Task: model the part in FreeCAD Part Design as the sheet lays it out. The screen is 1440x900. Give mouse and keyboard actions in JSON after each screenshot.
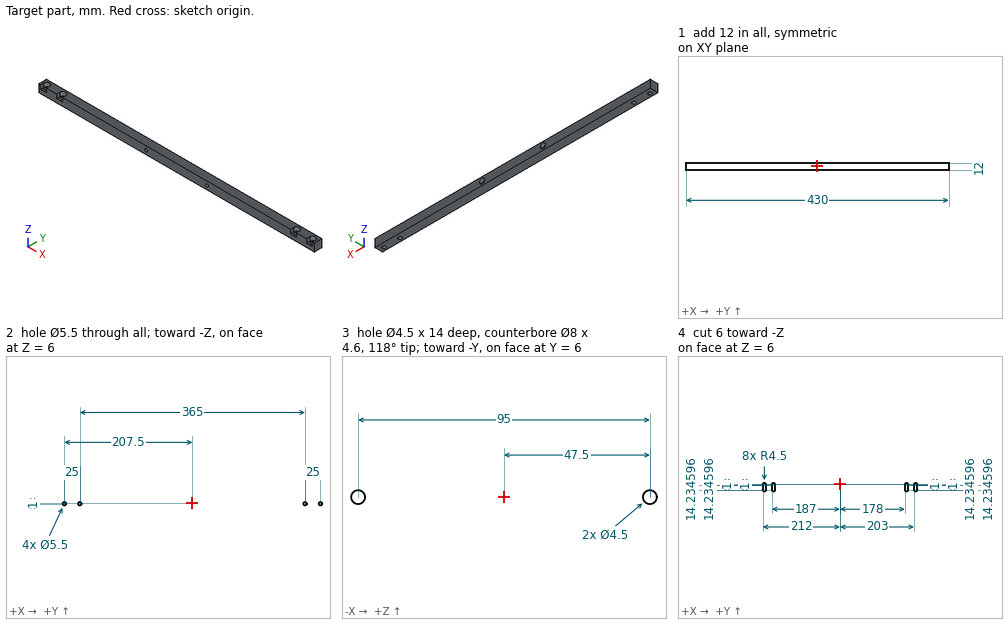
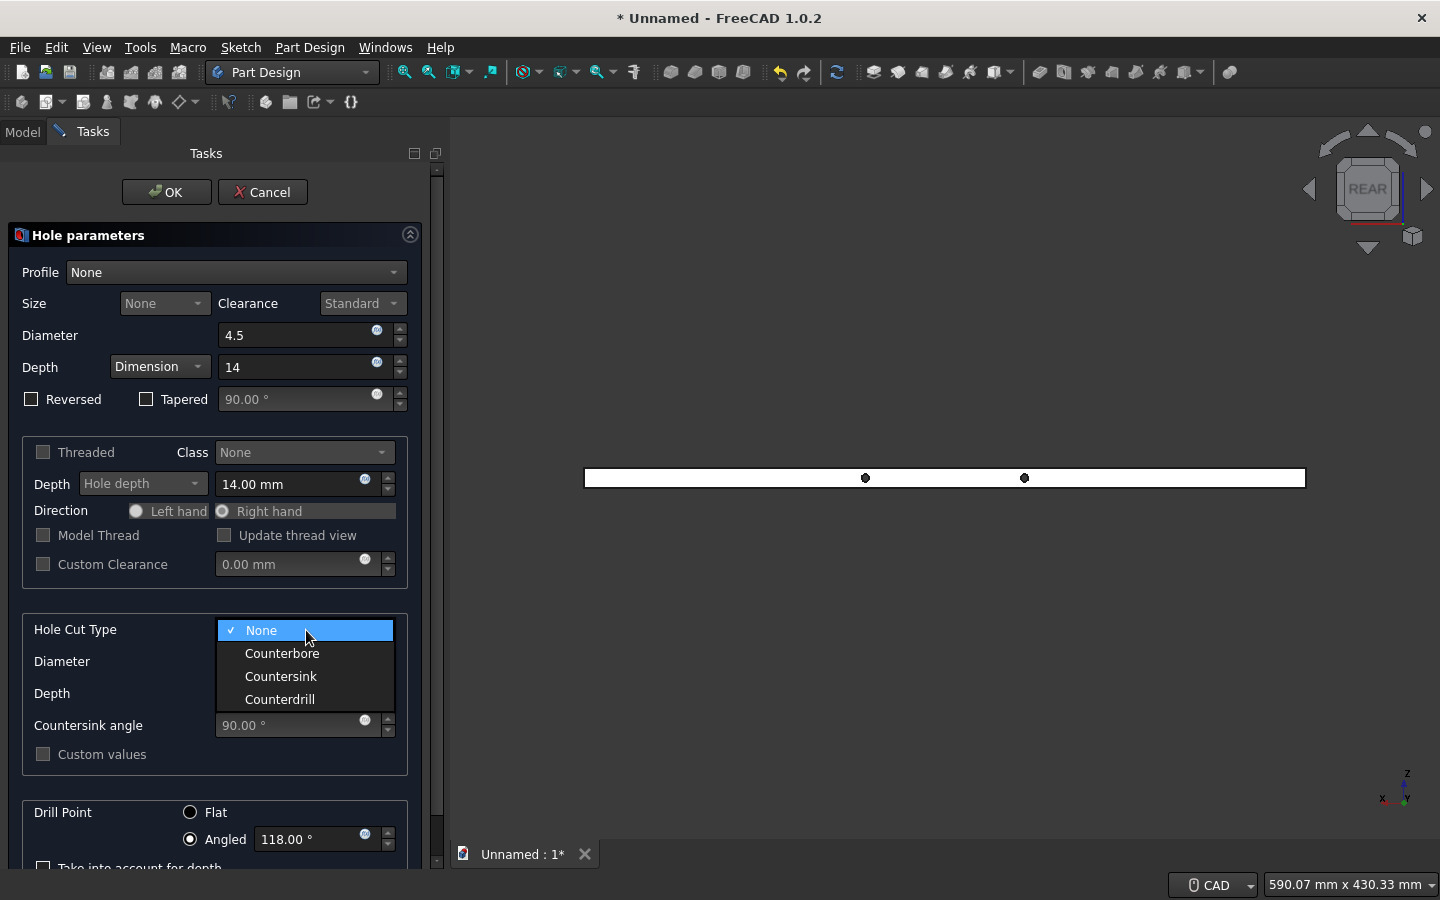
{"action": "left_click", "coordinate": [304, 654]}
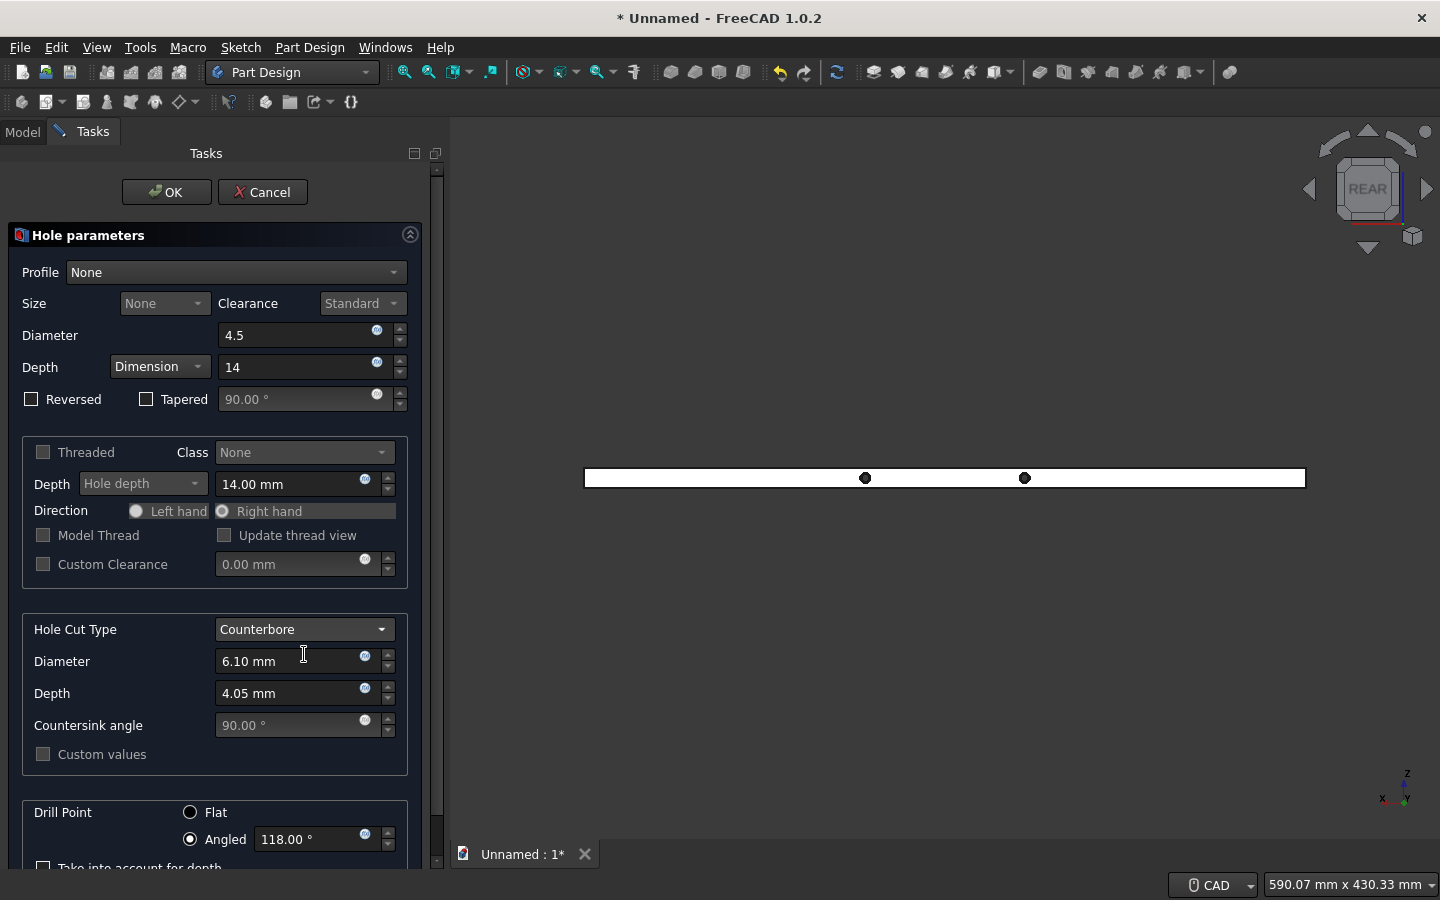
{"action": "triple_click", "coordinate": [298, 661]}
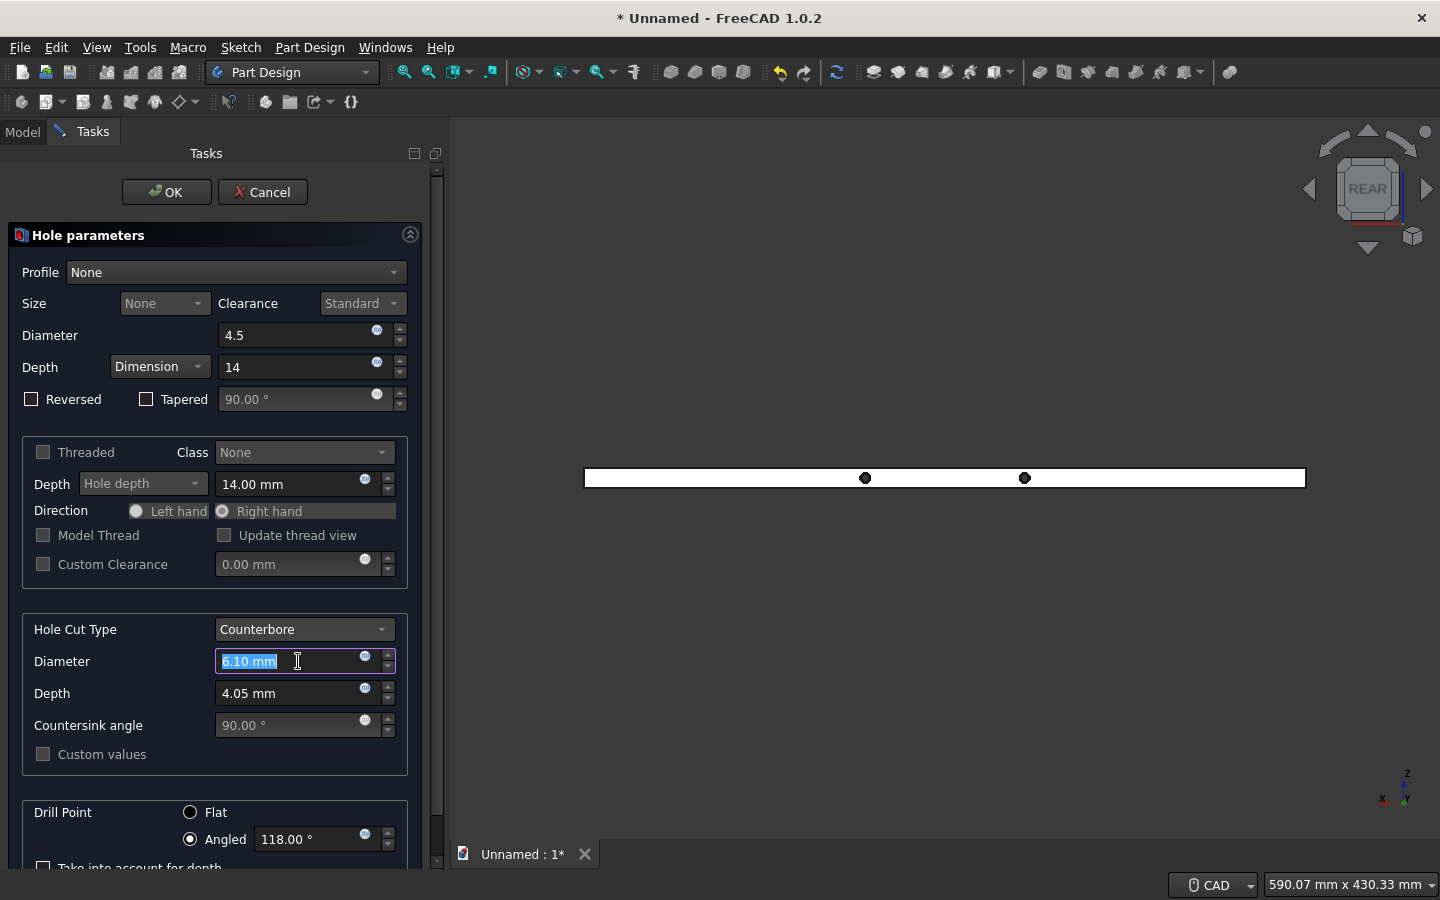
{"action": "type", "text": "8"}
{"action": "key", "text": "Tab"}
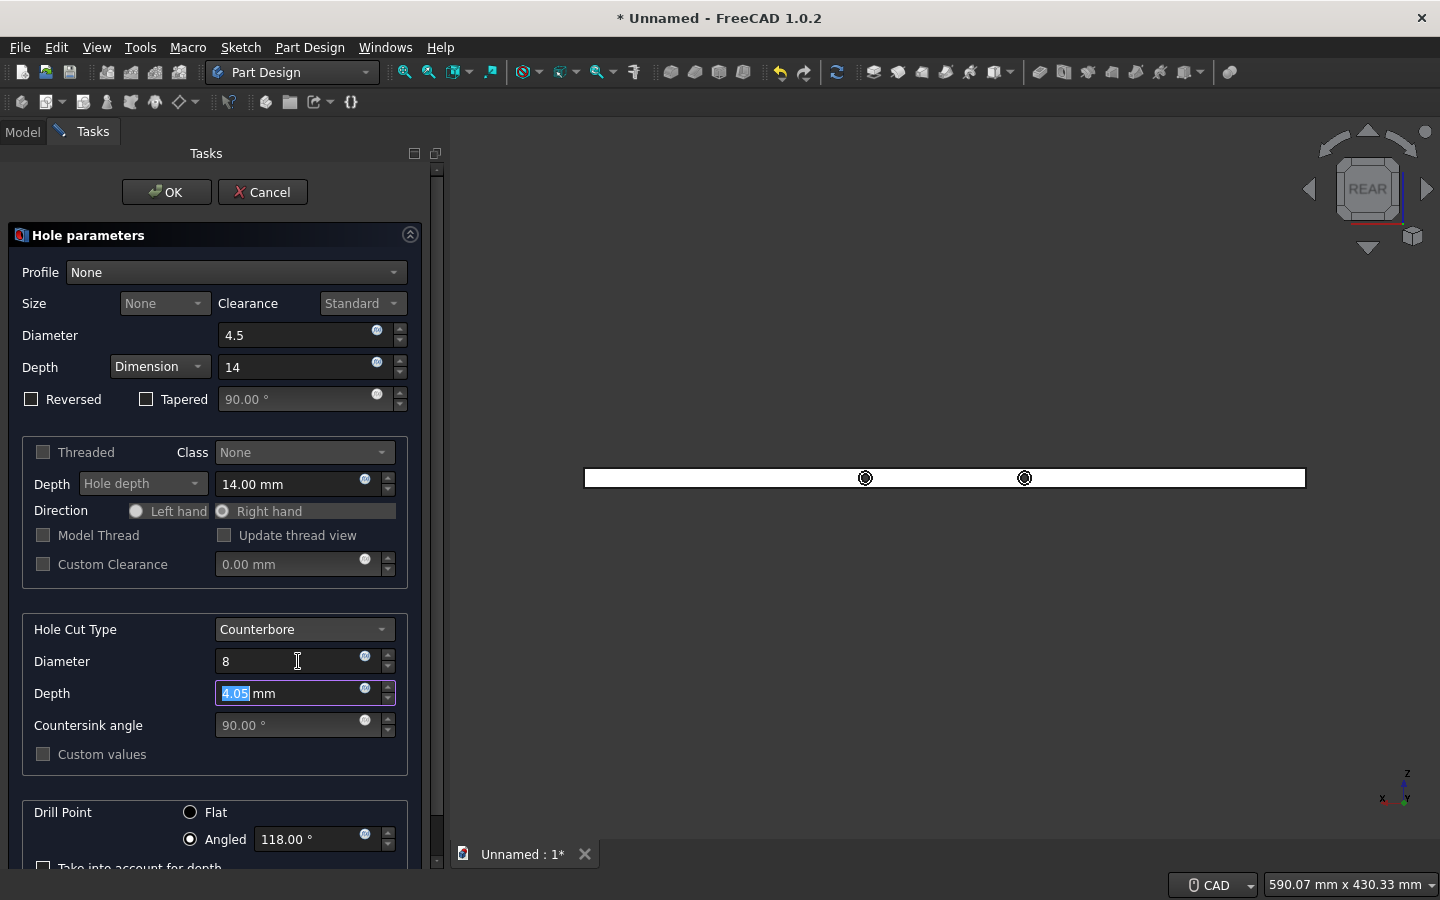
{"action": "type", "text": "4.6"}
{"action": "key", "text": "Tab"}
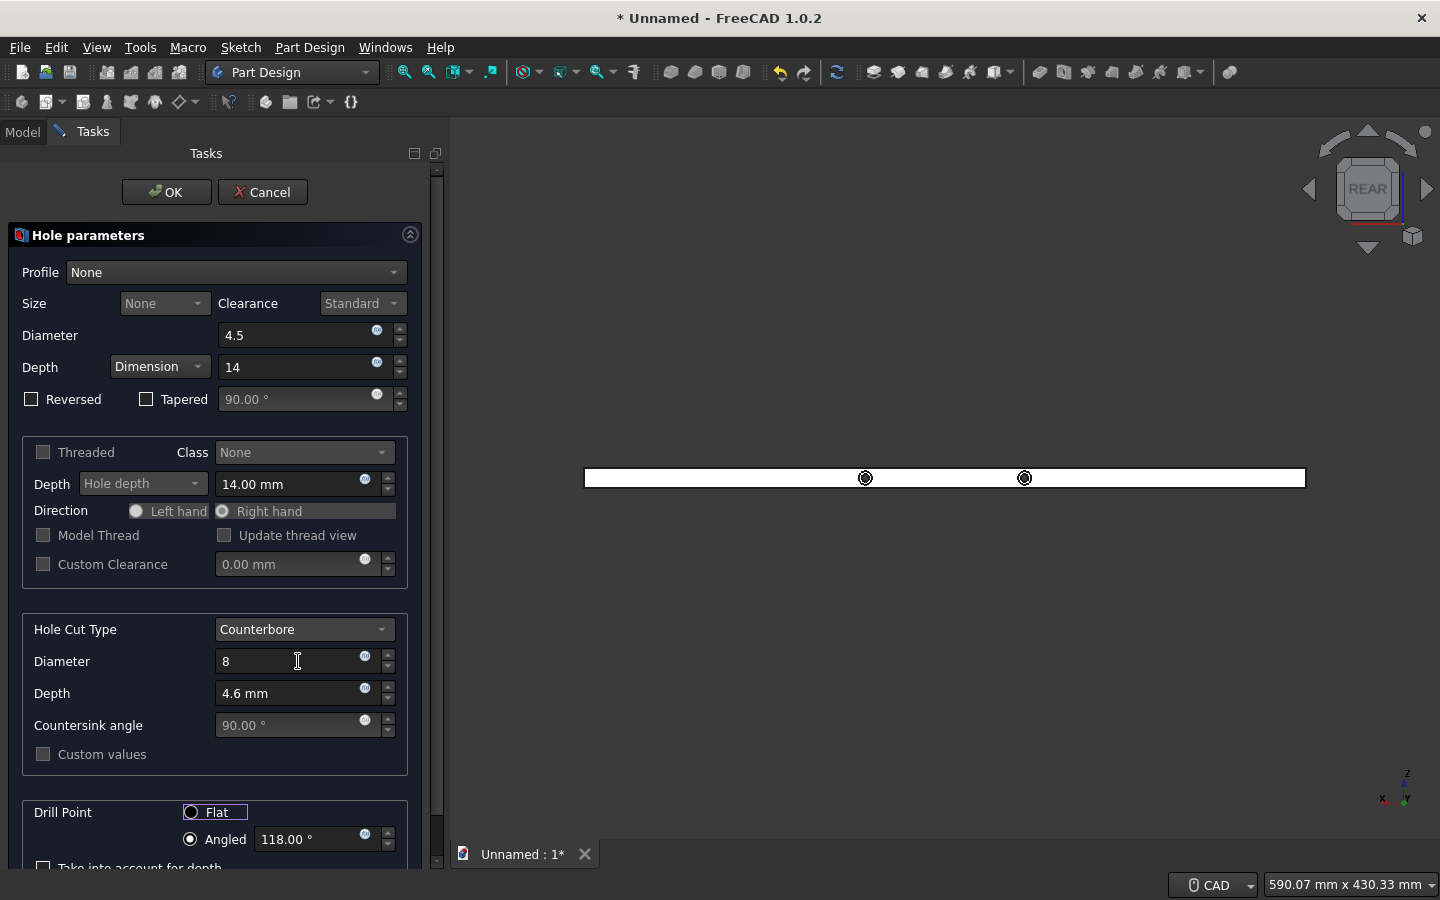
{"action": "left_click", "coordinate": [167, 192]}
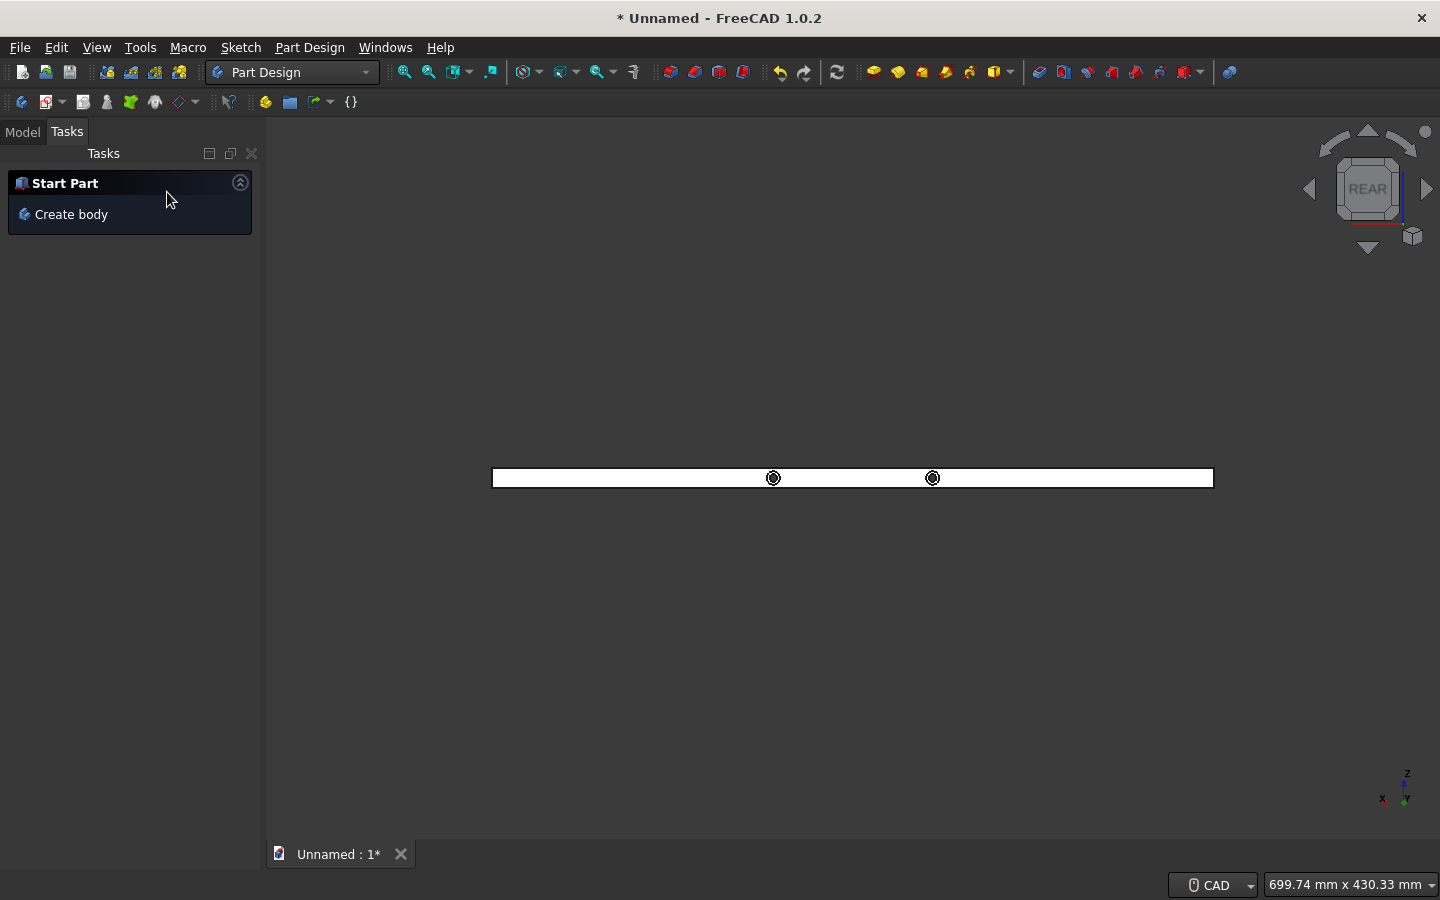
{"action": "key", "text": "0"}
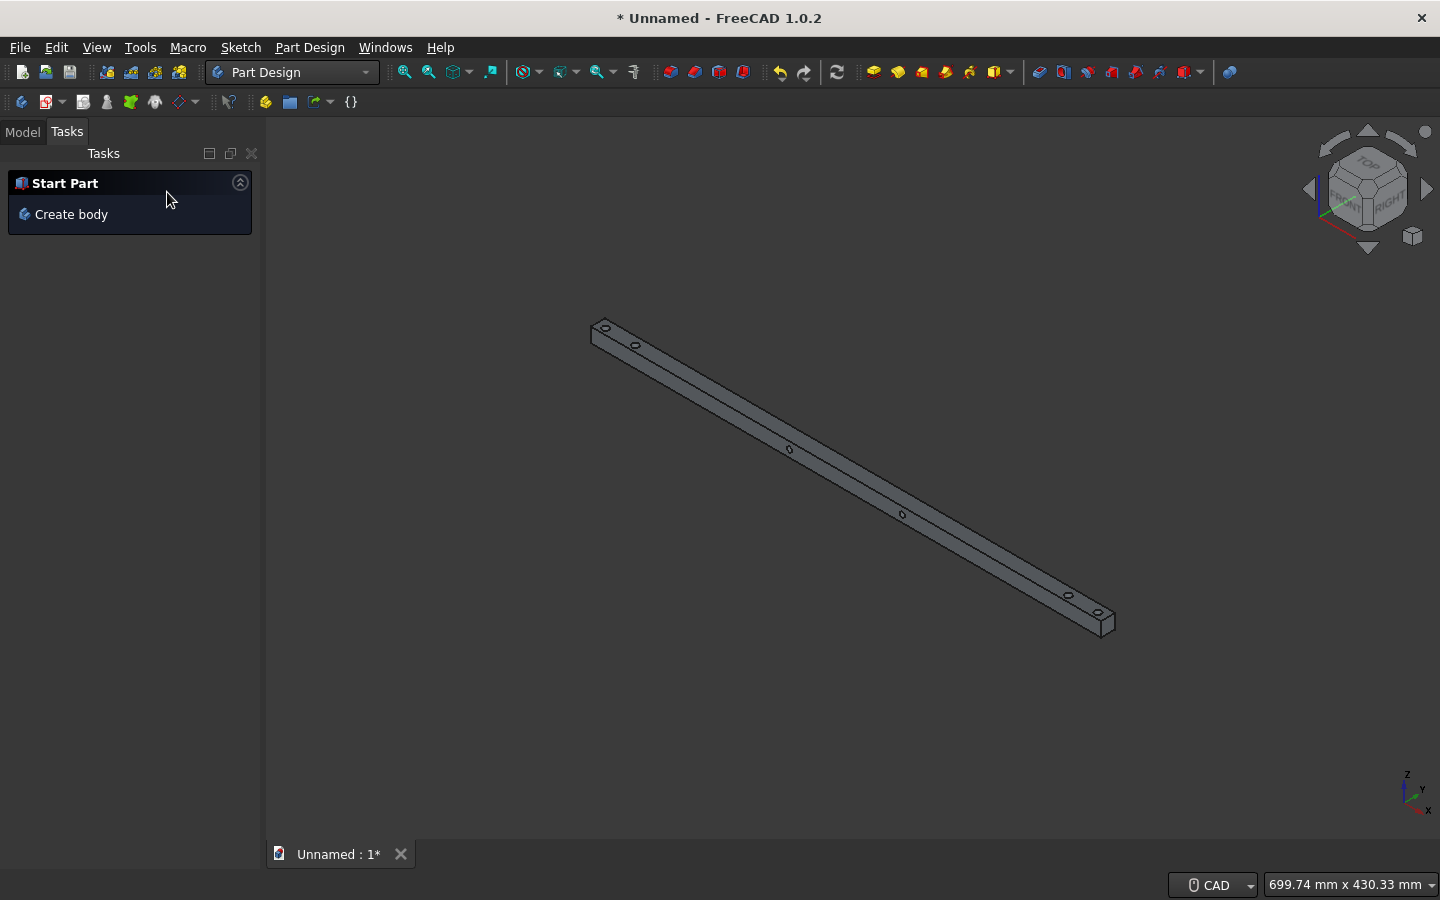
{"action": "left_click", "coordinate": [406, 72]}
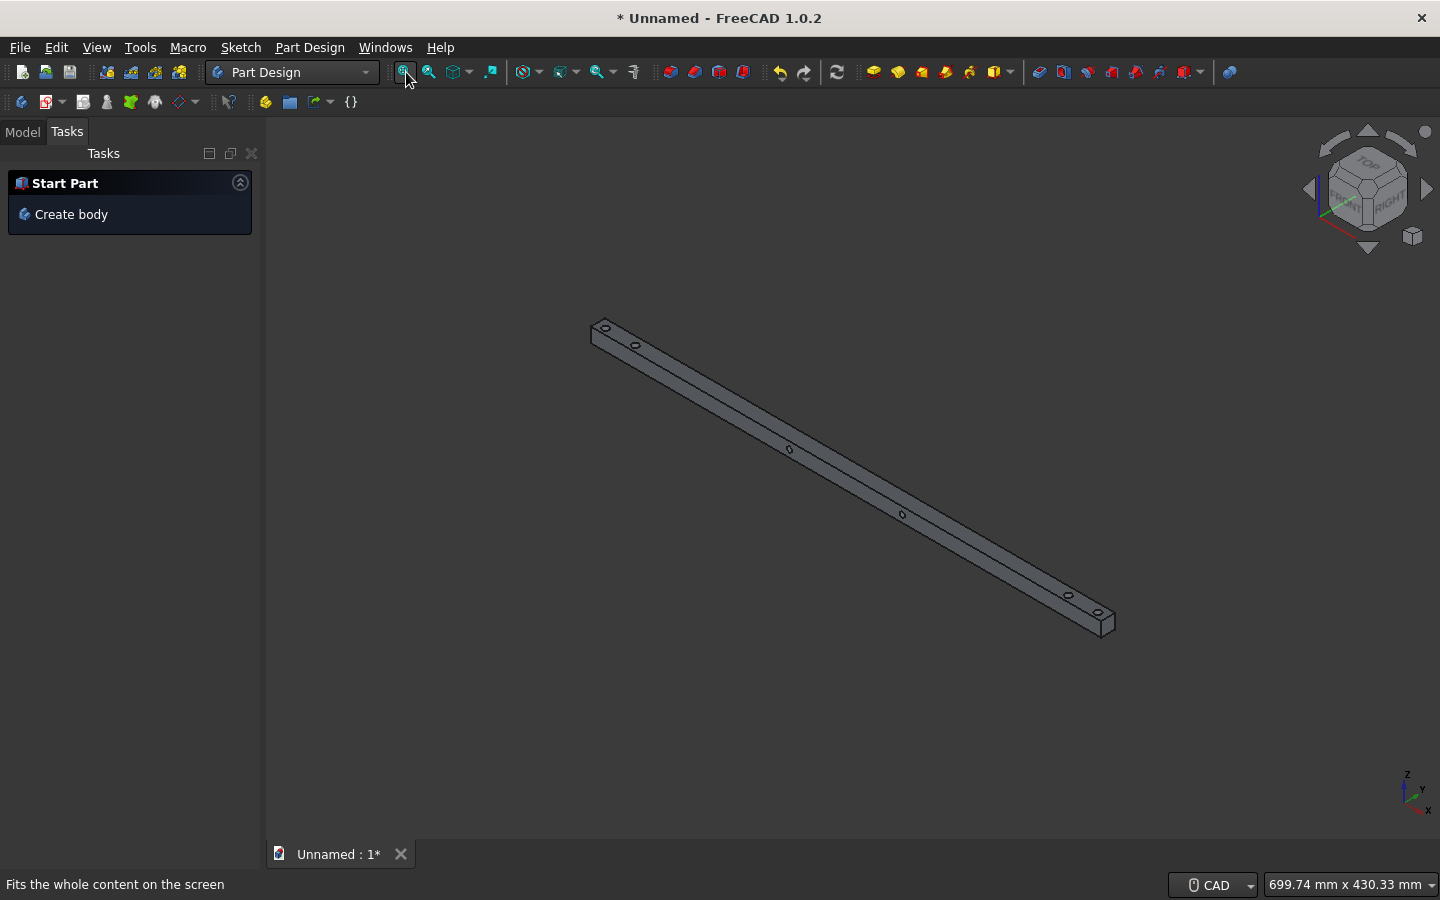
{"action": "key", "text": "2"}